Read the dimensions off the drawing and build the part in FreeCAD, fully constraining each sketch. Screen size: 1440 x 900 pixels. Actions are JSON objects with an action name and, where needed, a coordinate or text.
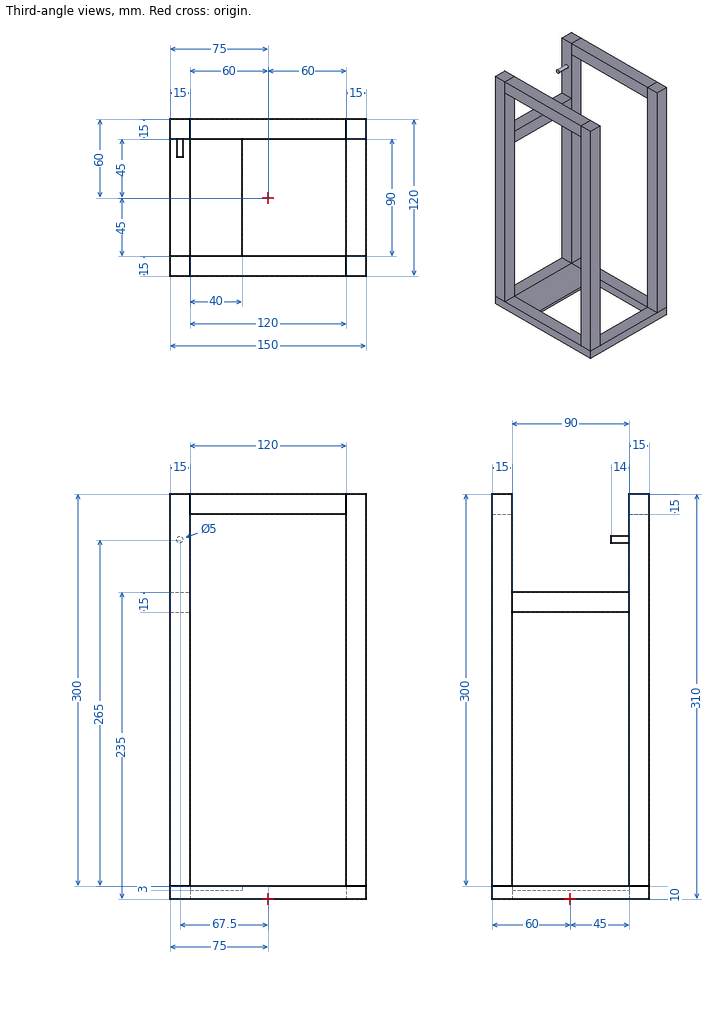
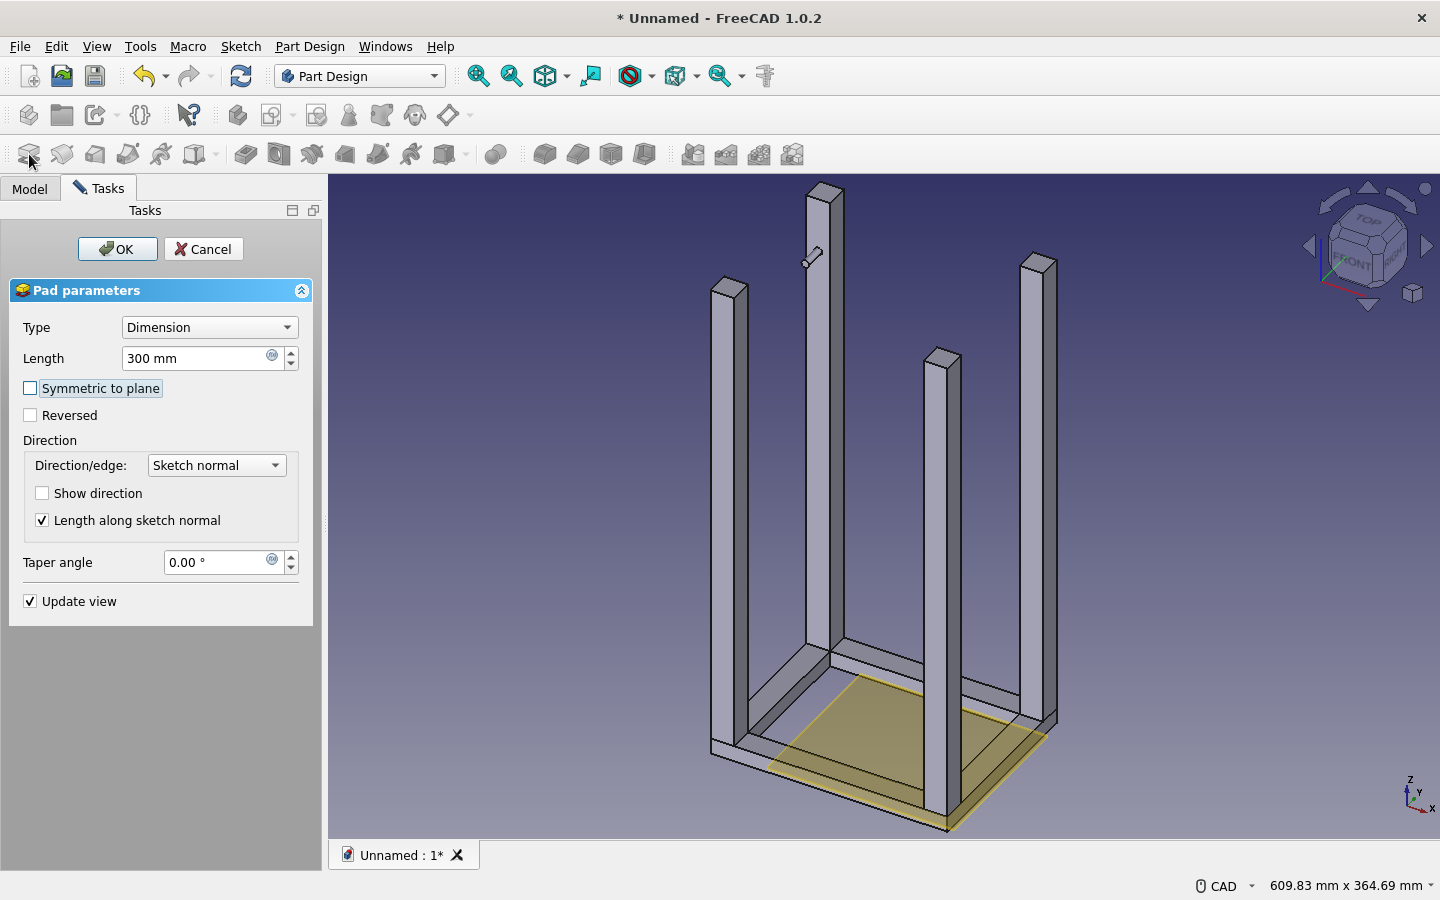
{"action": "left_click", "coordinate": [118, 249]}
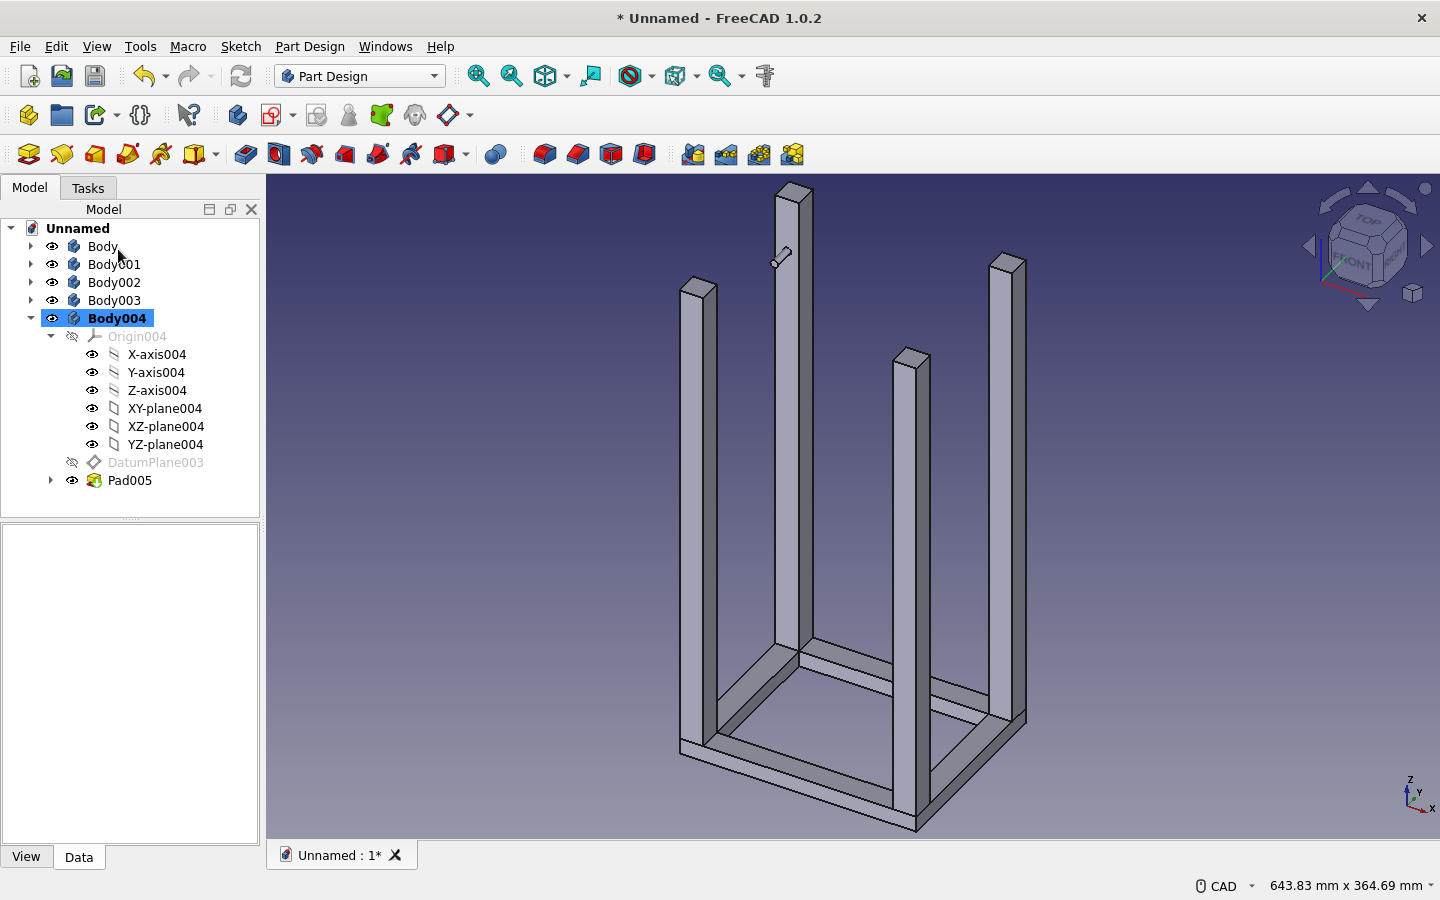
{"action": "left_click", "coordinate": [238, 116]}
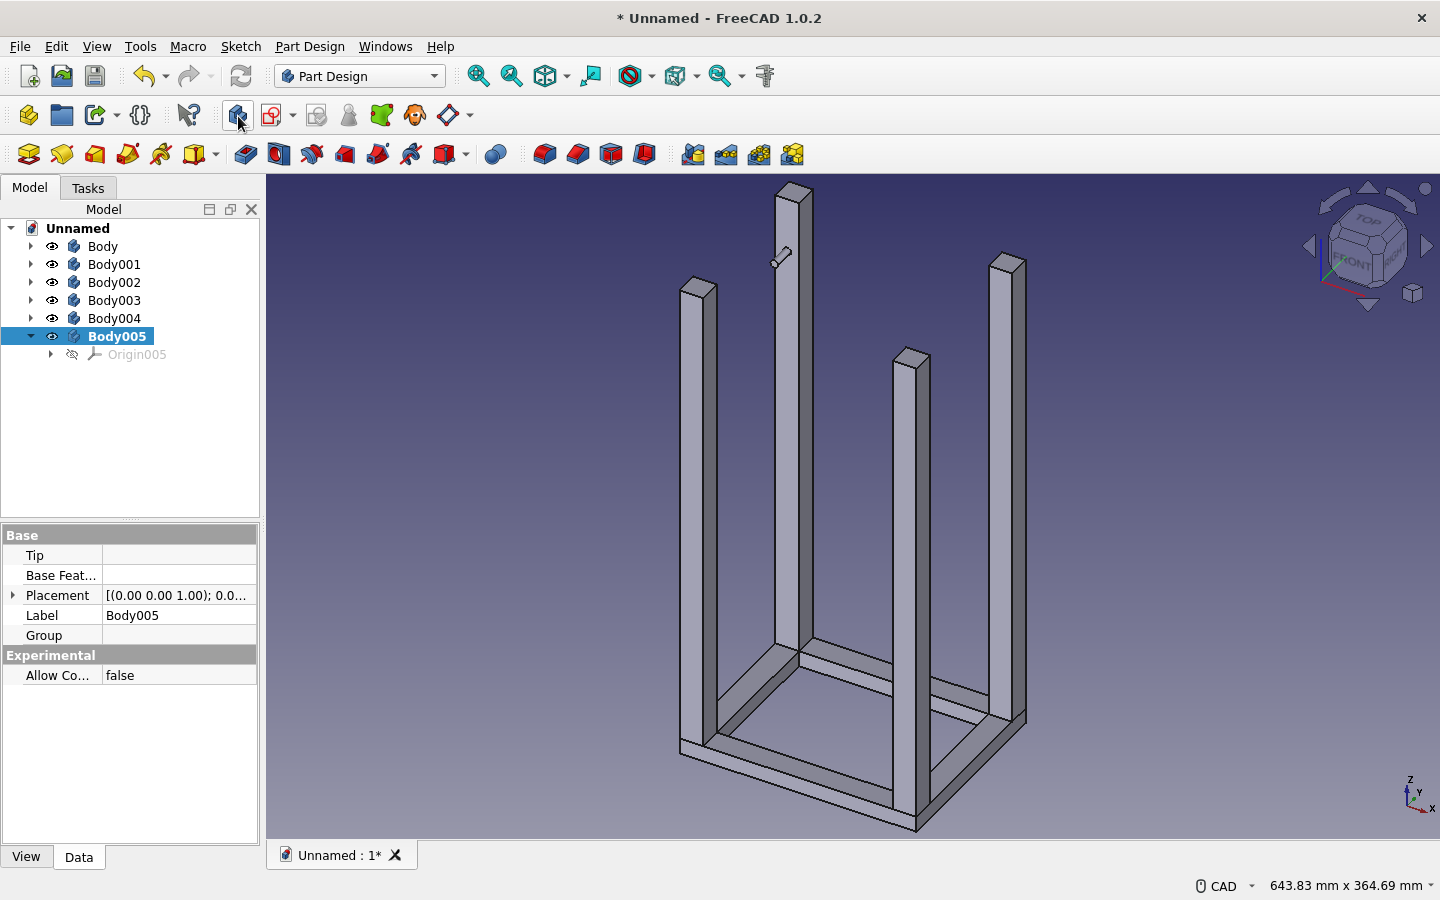
{"action": "left_click", "coordinate": [51, 354]}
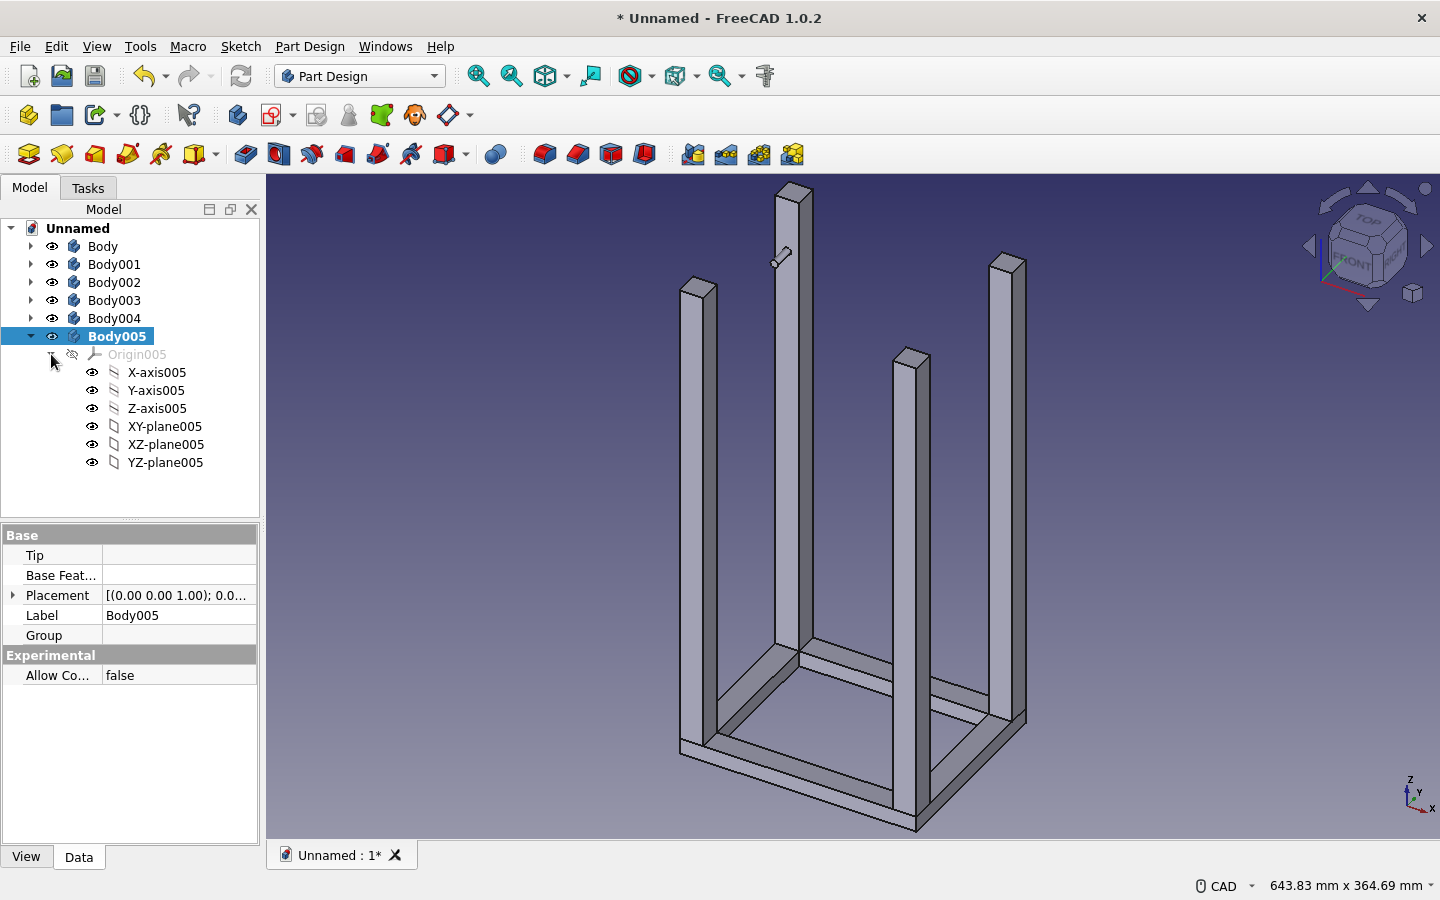
{"action": "left_click", "coordinate": [137, 462]}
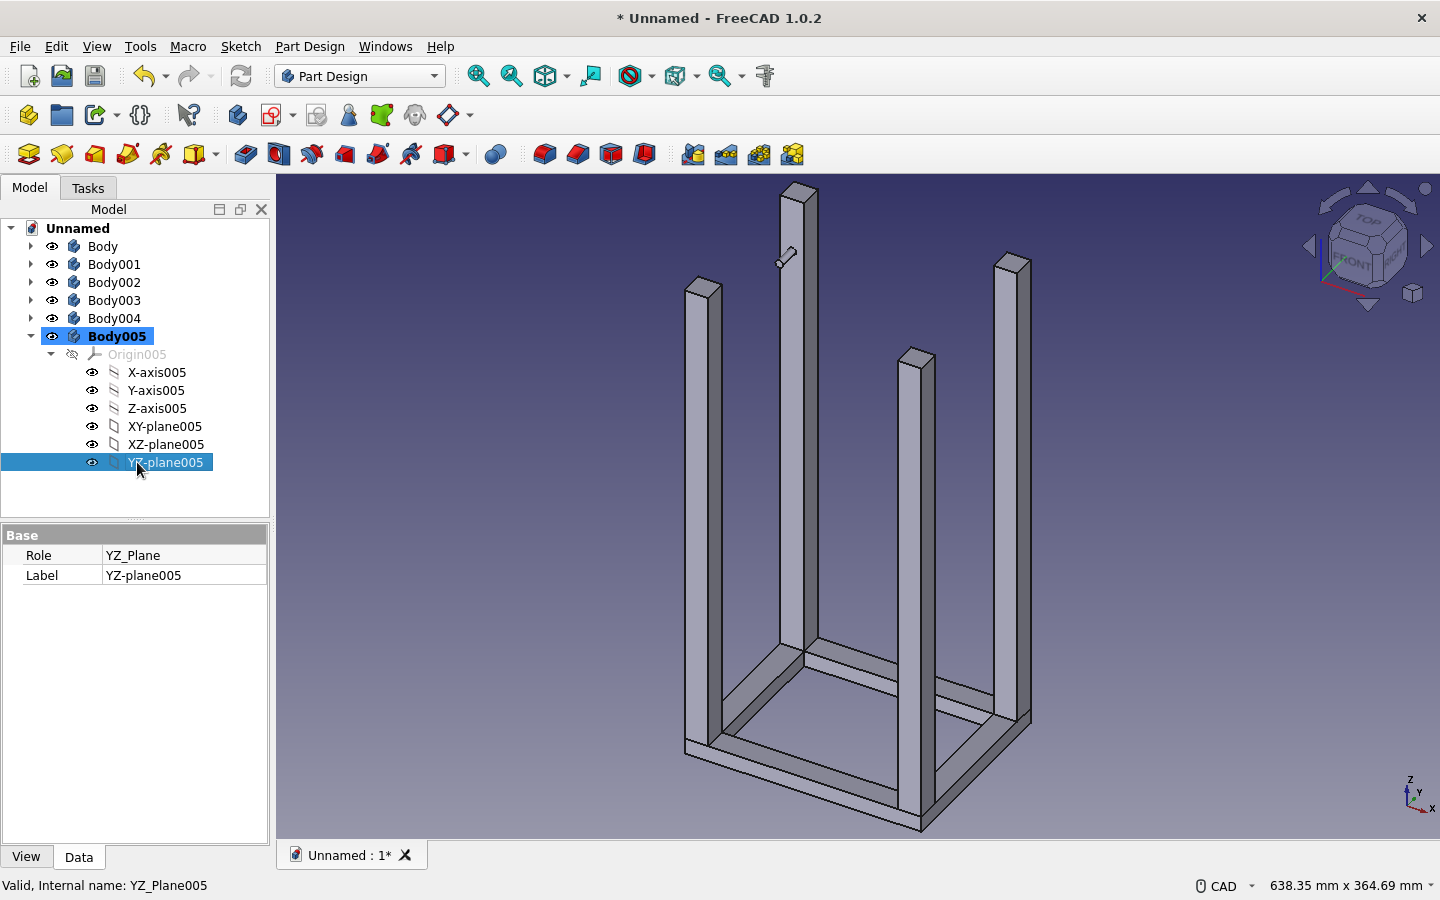
{"action": "left_click", "coordinate": [448, 116]}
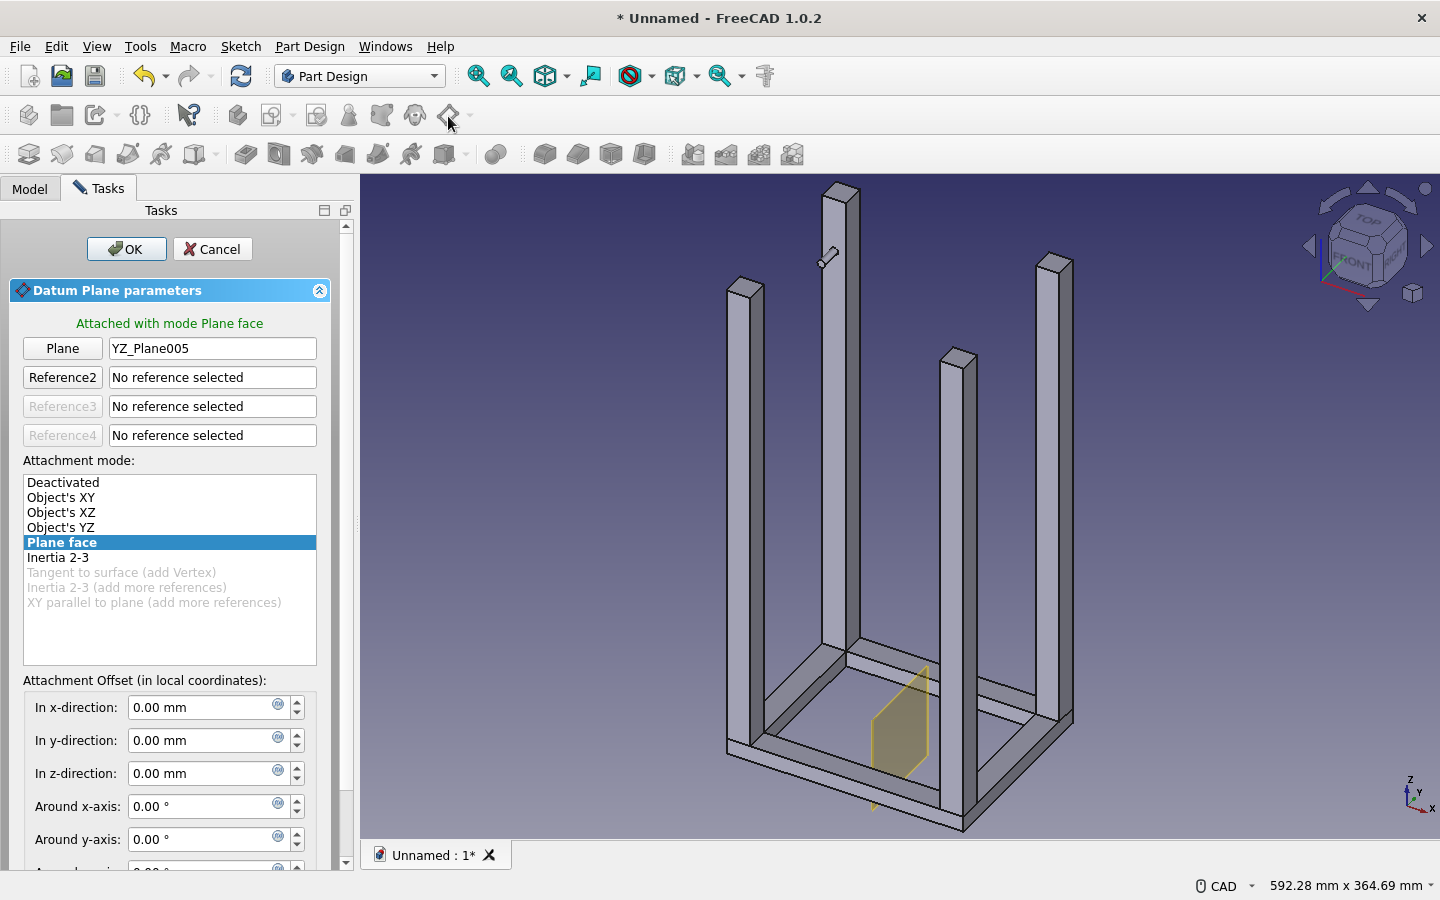
{"action": "triple_click", "coordinate": [210, 774]}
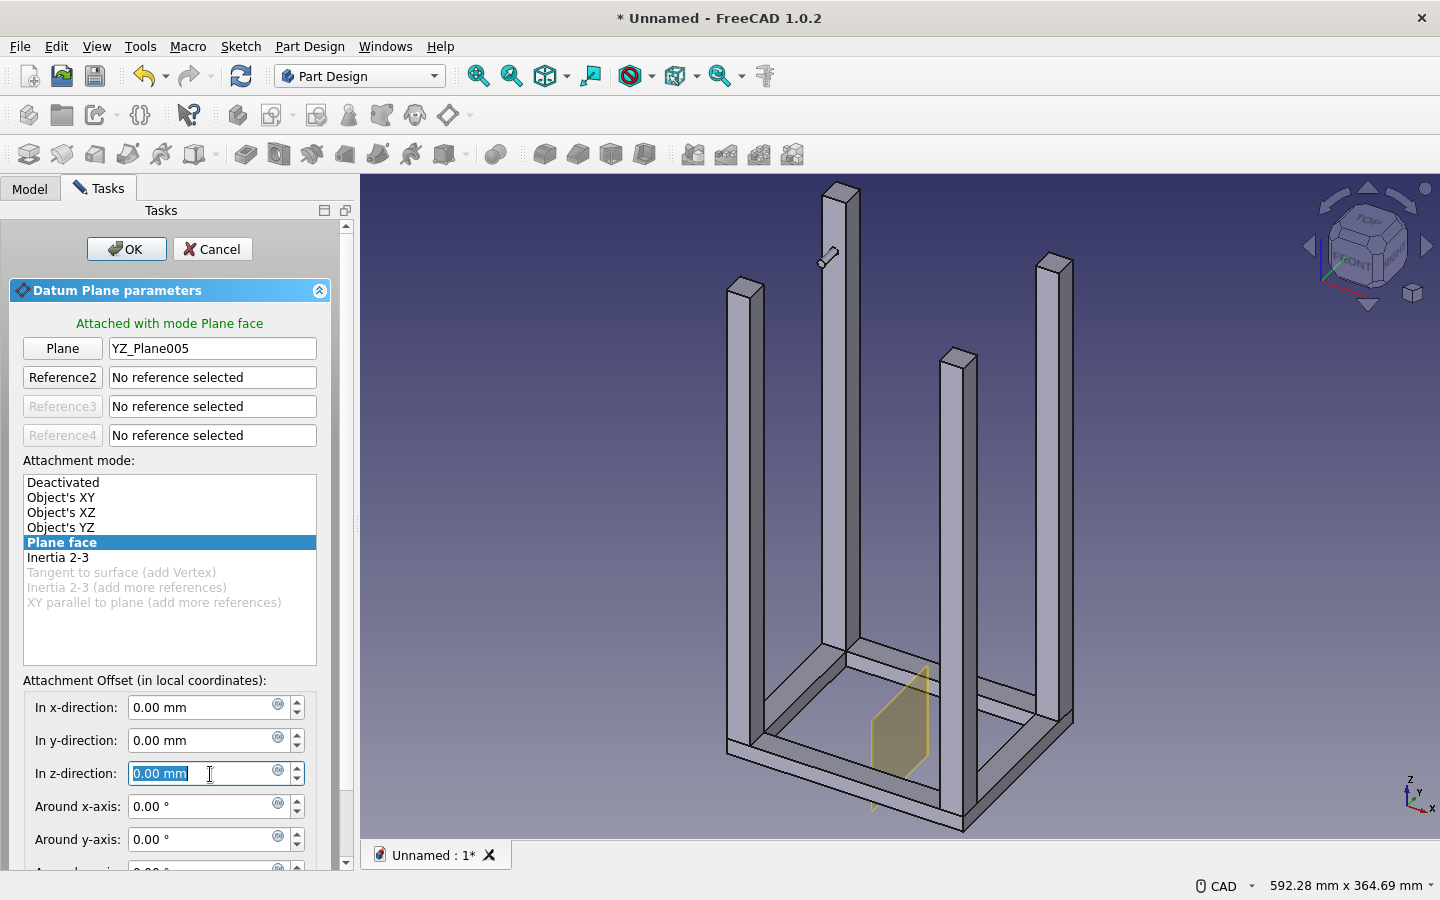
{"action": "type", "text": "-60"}
{"action": "key", "text": "Tab"}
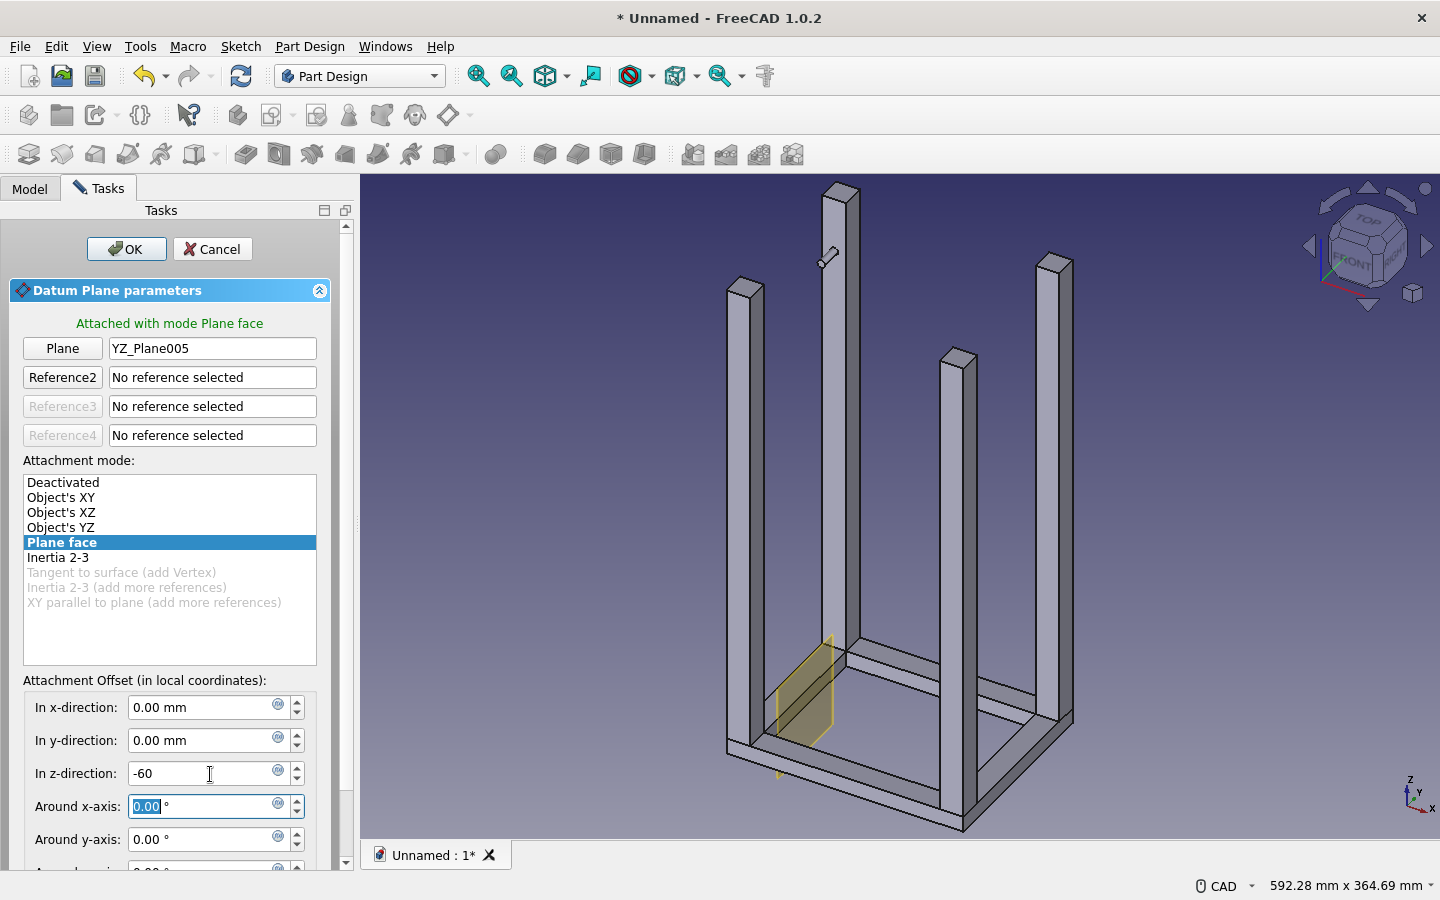
{"action": "left_click", "coordinate": [127, 249]}